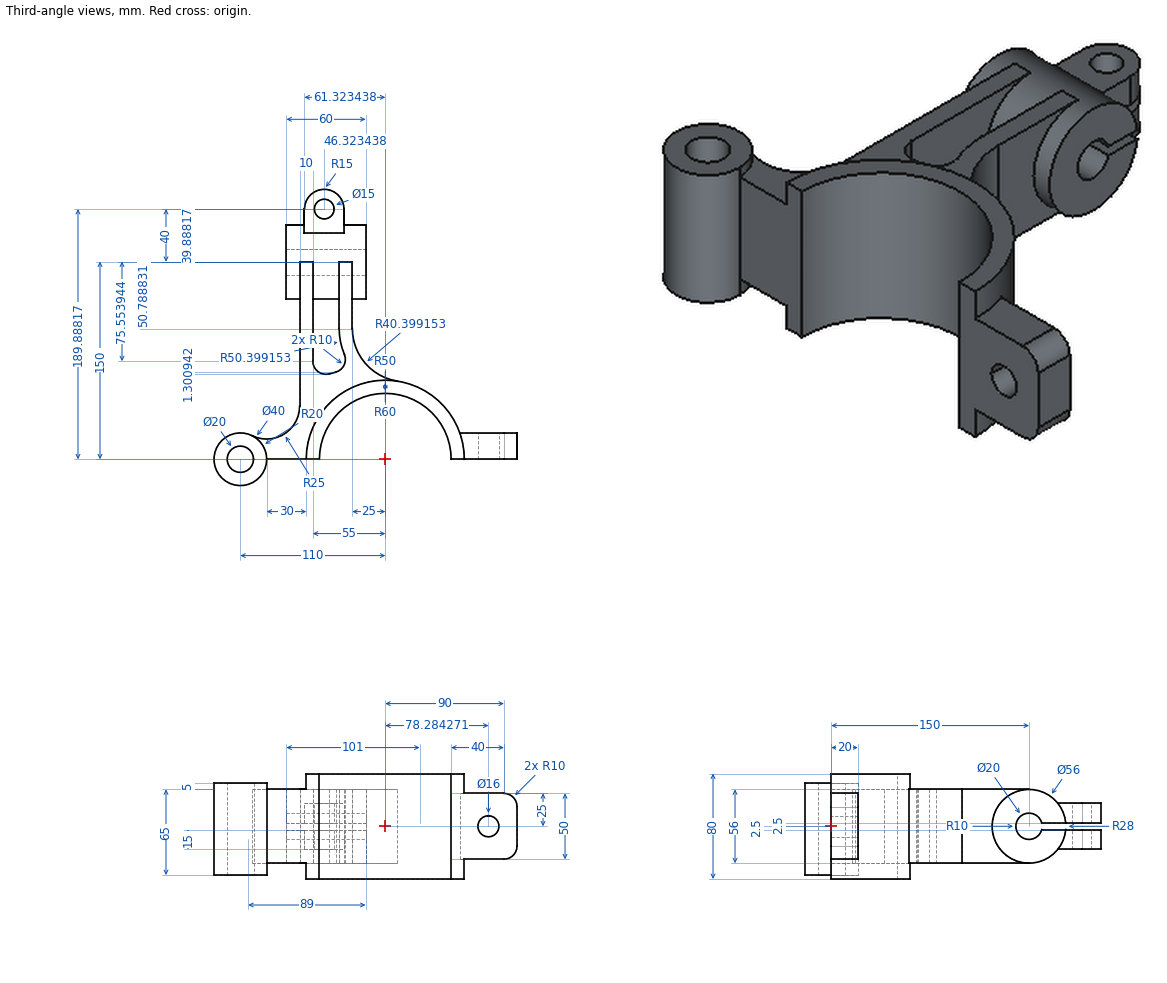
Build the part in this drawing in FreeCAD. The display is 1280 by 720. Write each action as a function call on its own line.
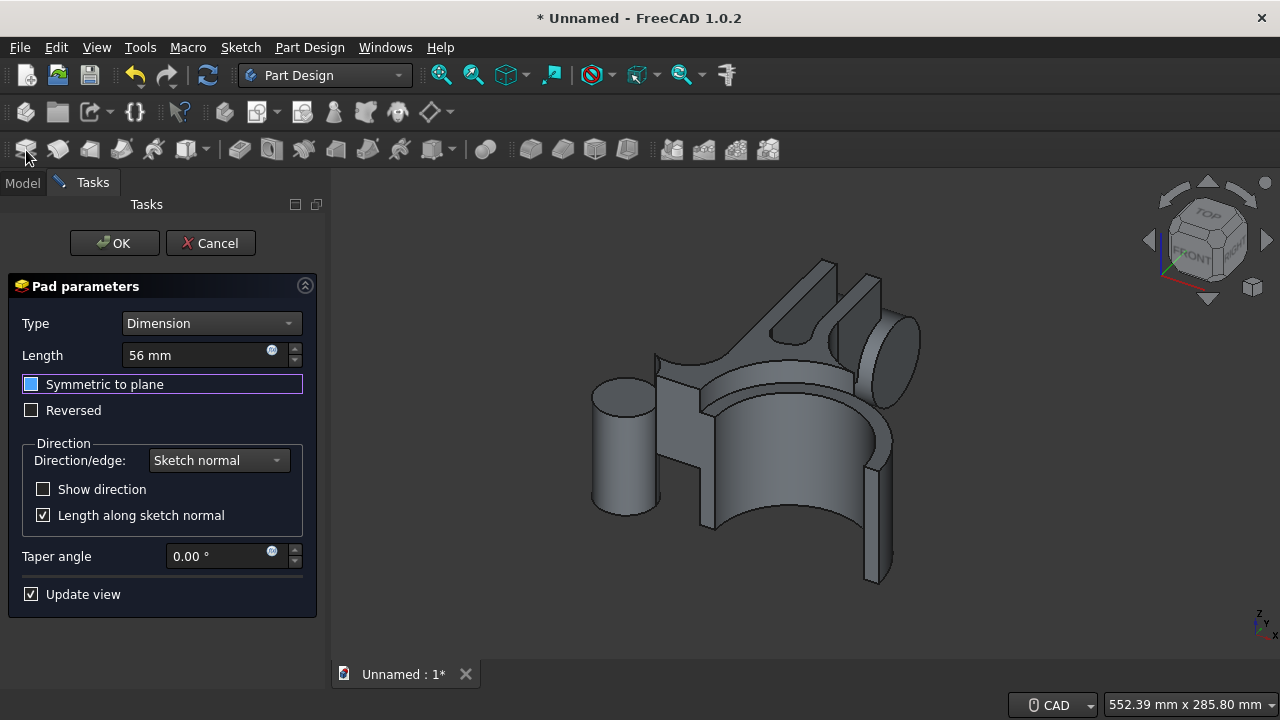
click(30, 384)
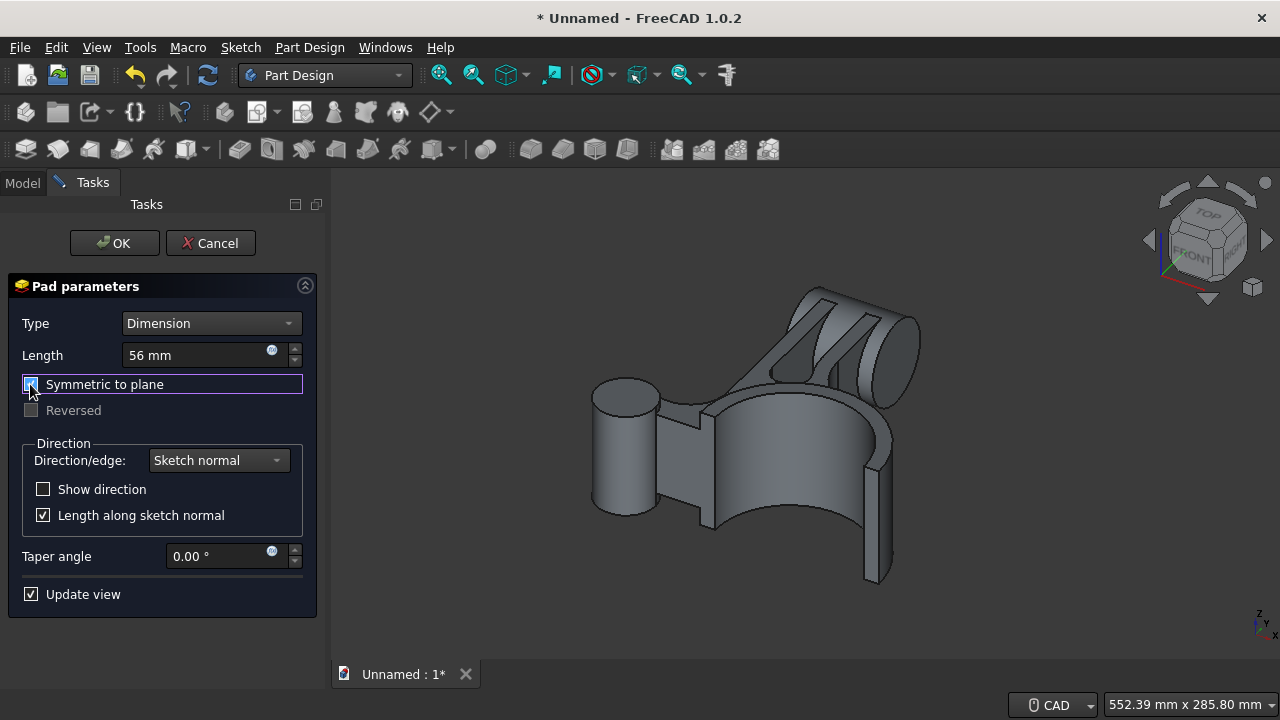
click(115, 243)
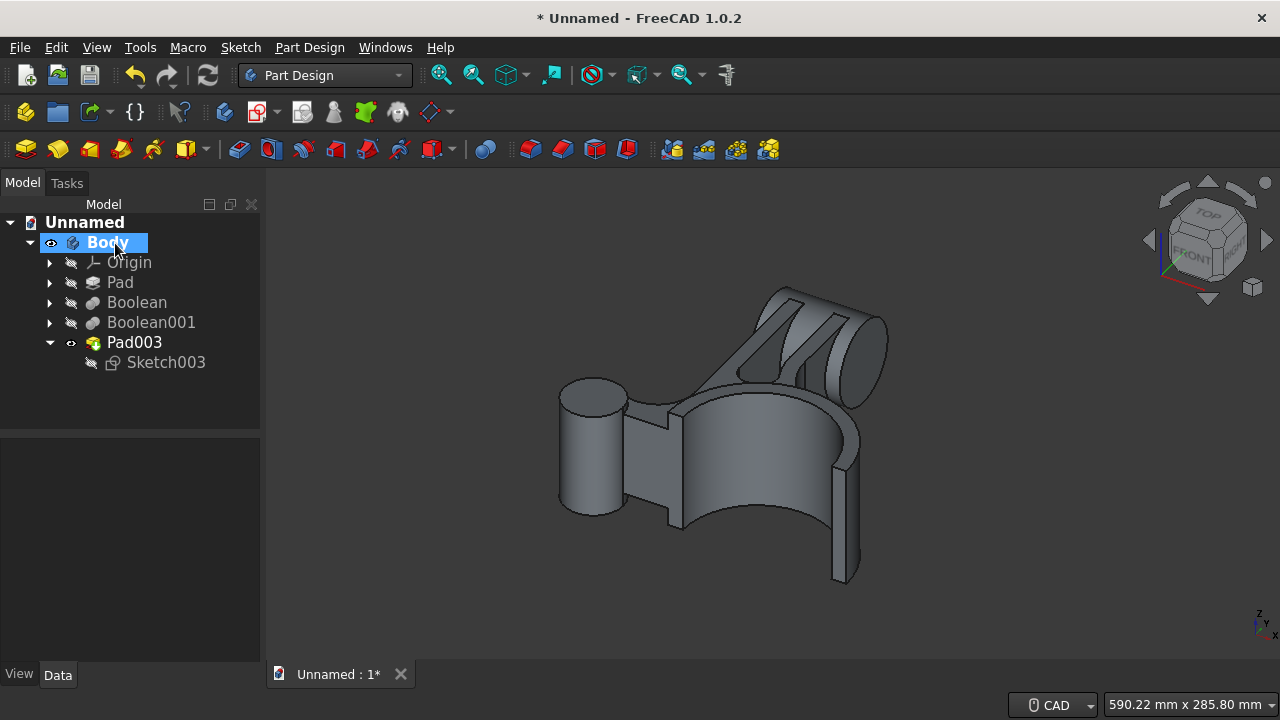
click(50, 263)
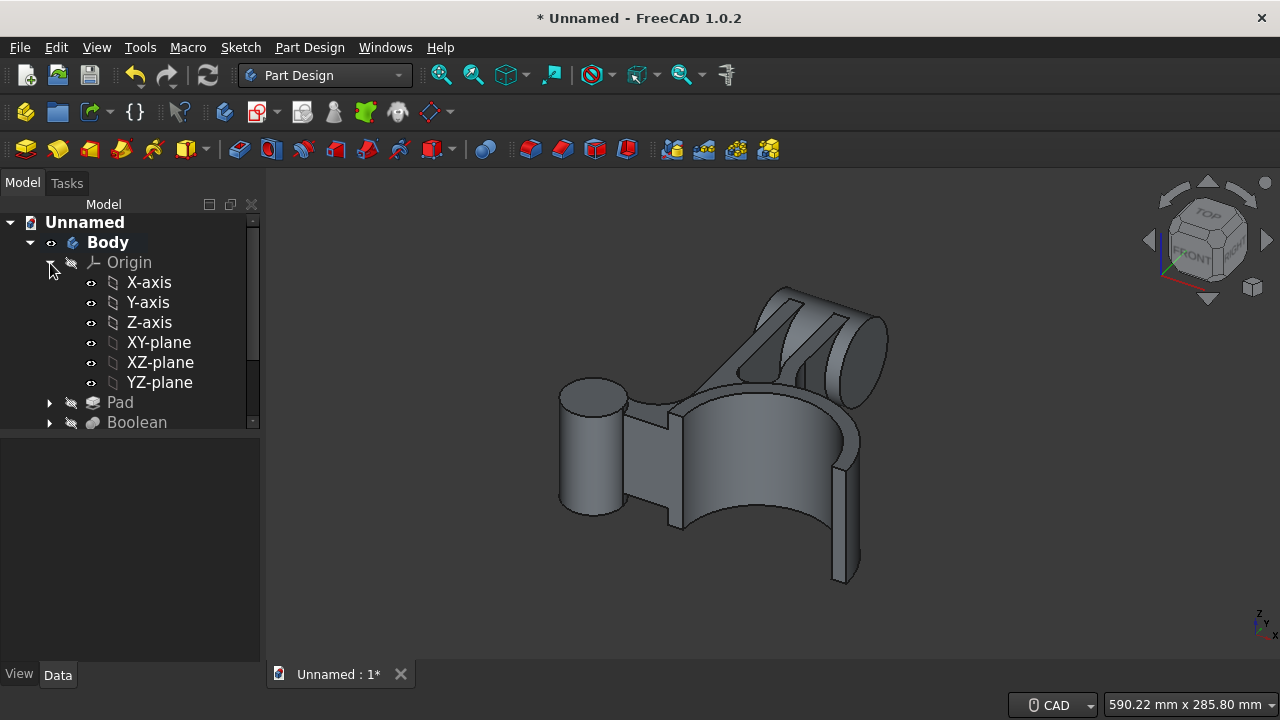
click(136, 383)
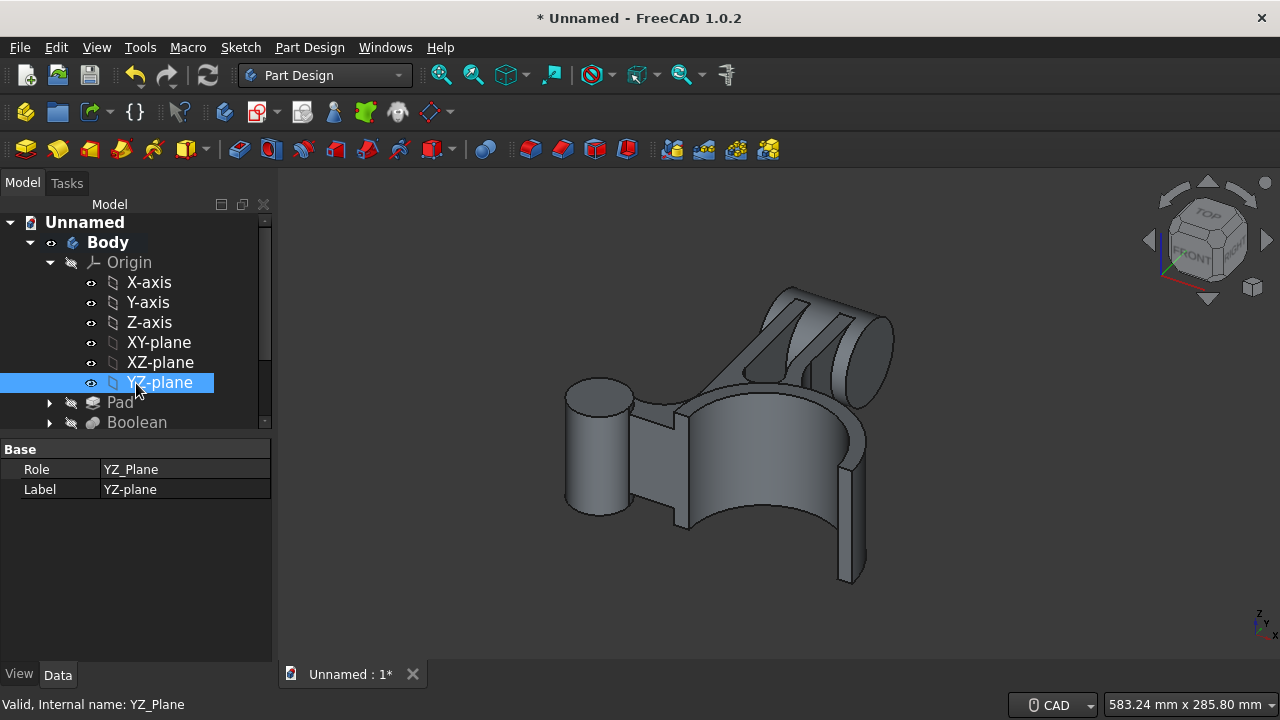
click(430, 112)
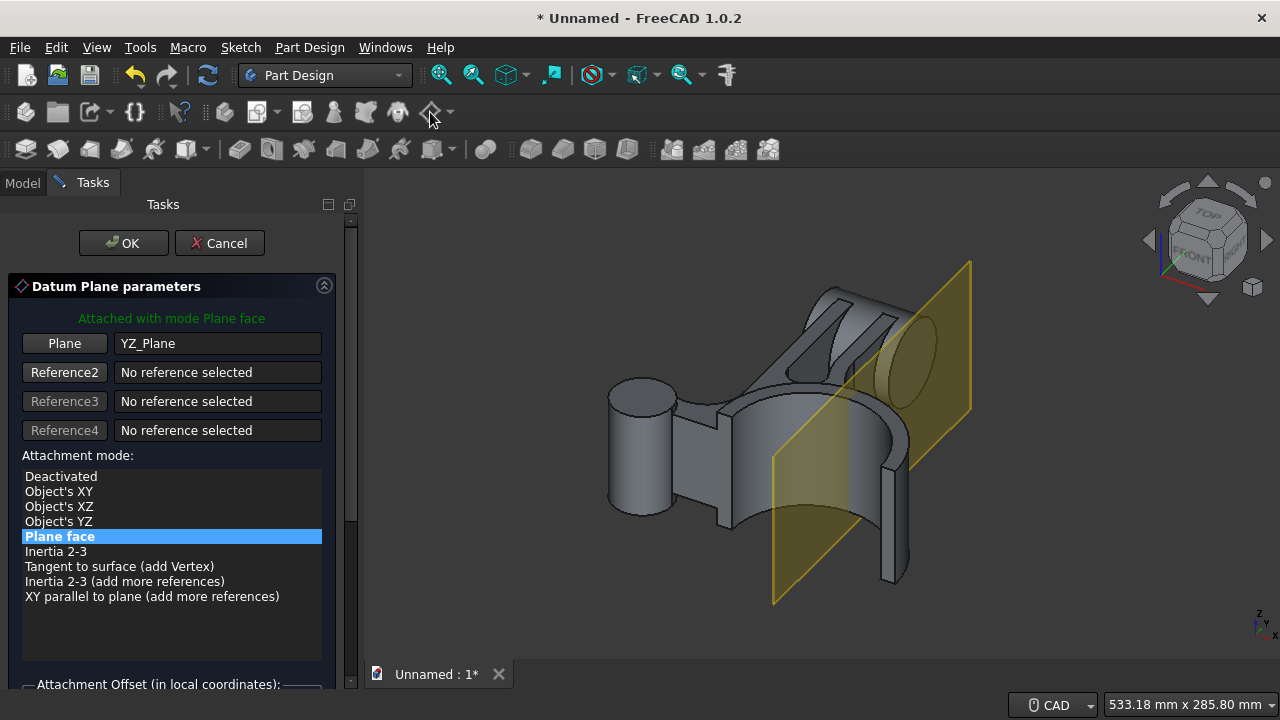
scroll(351, 451, down, 3)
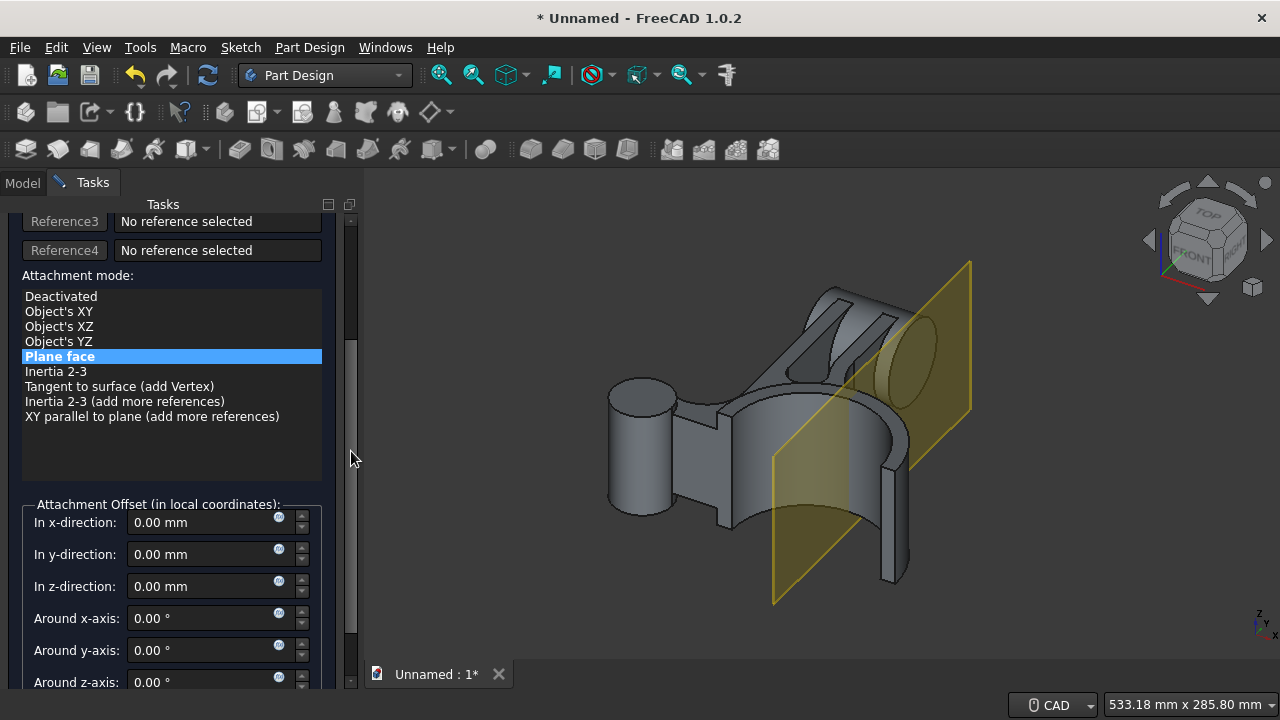
triple_click(210, 586)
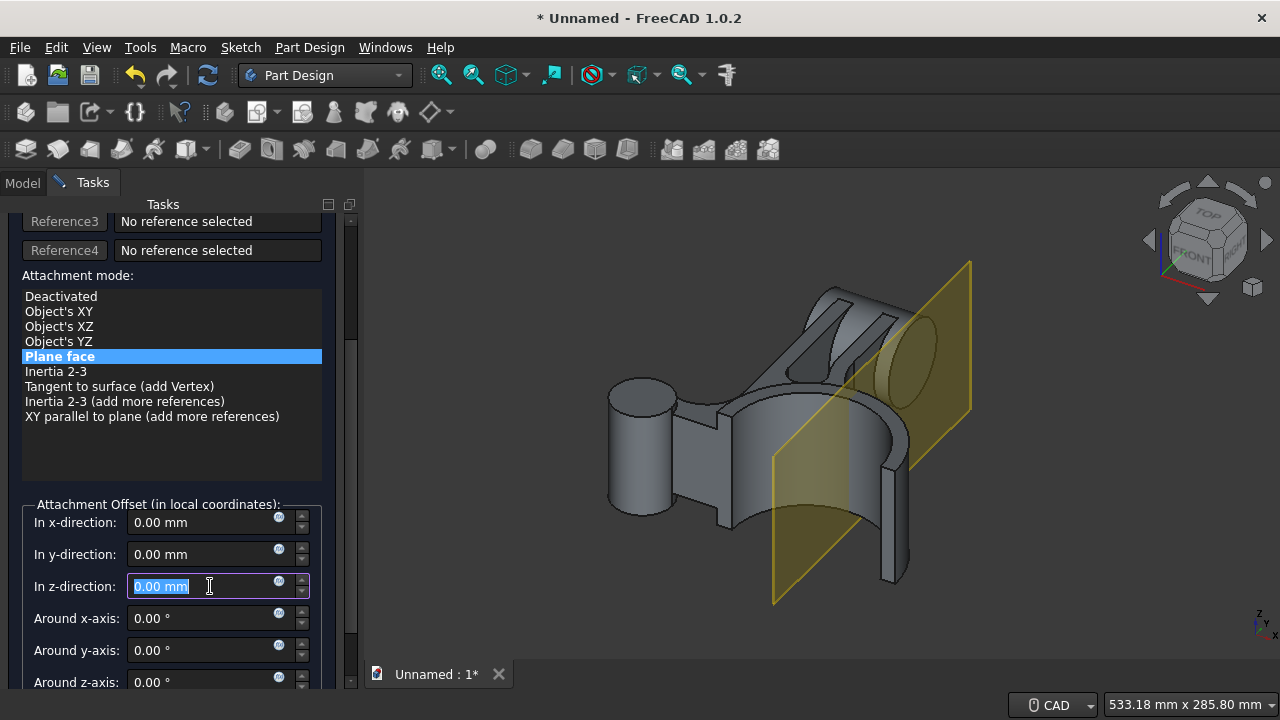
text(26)
key(Tab)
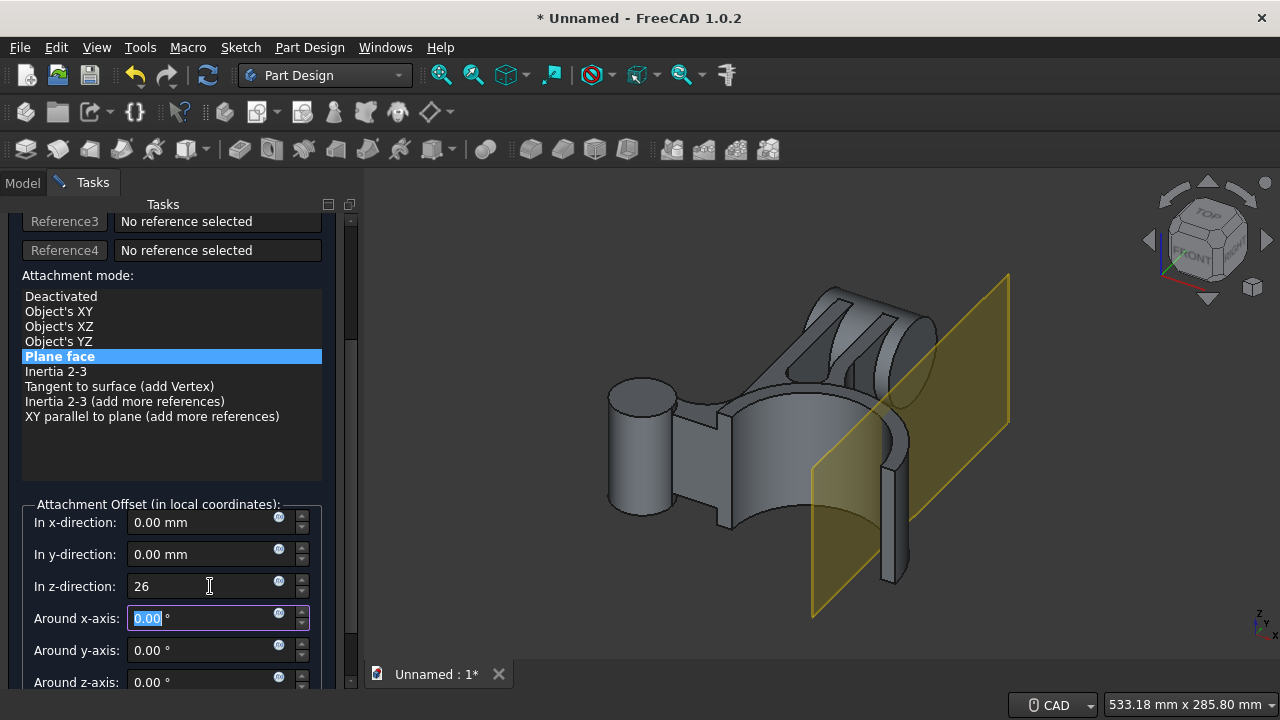
scroll(351, 451, up, 4)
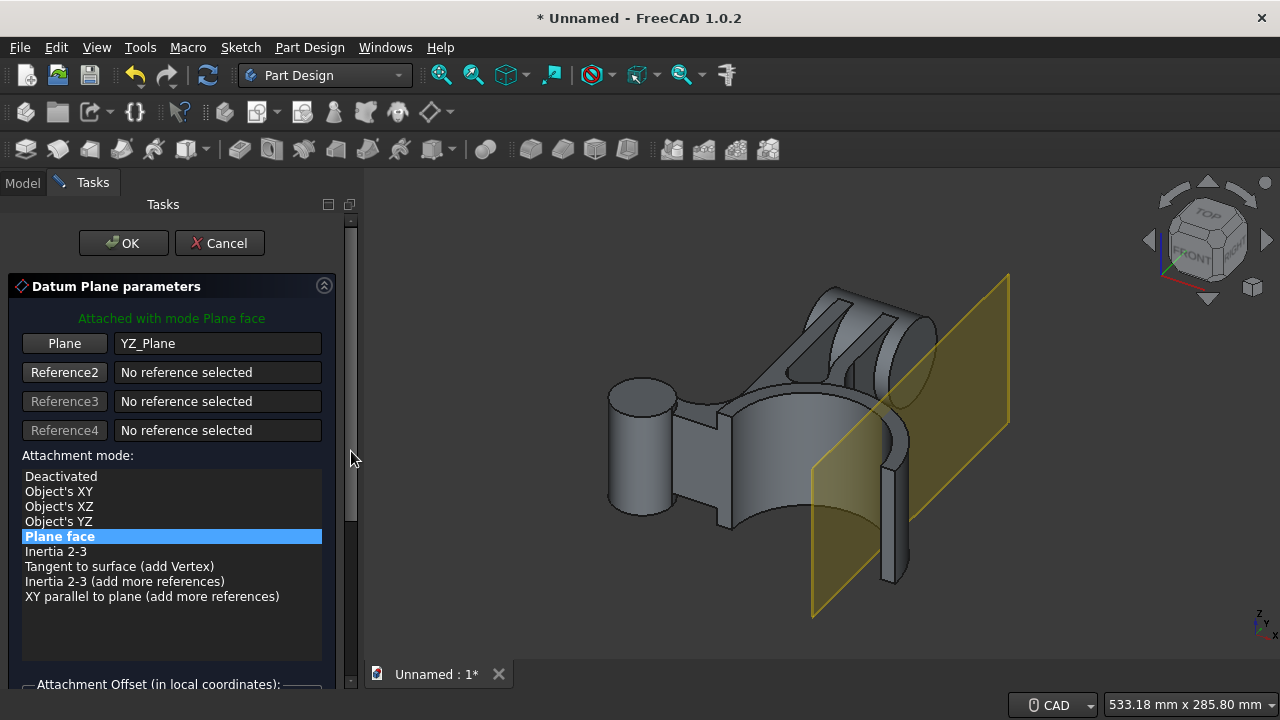
click(124, 243)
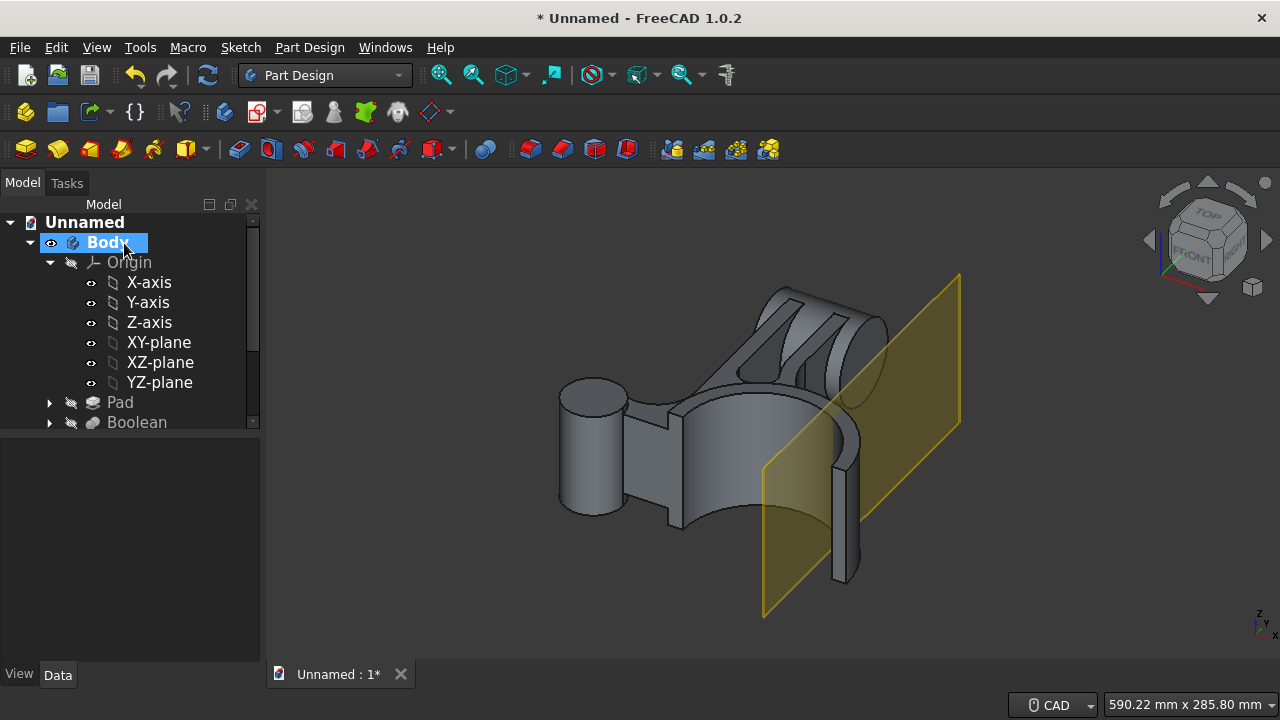
scroll(100, 318, down, 3)